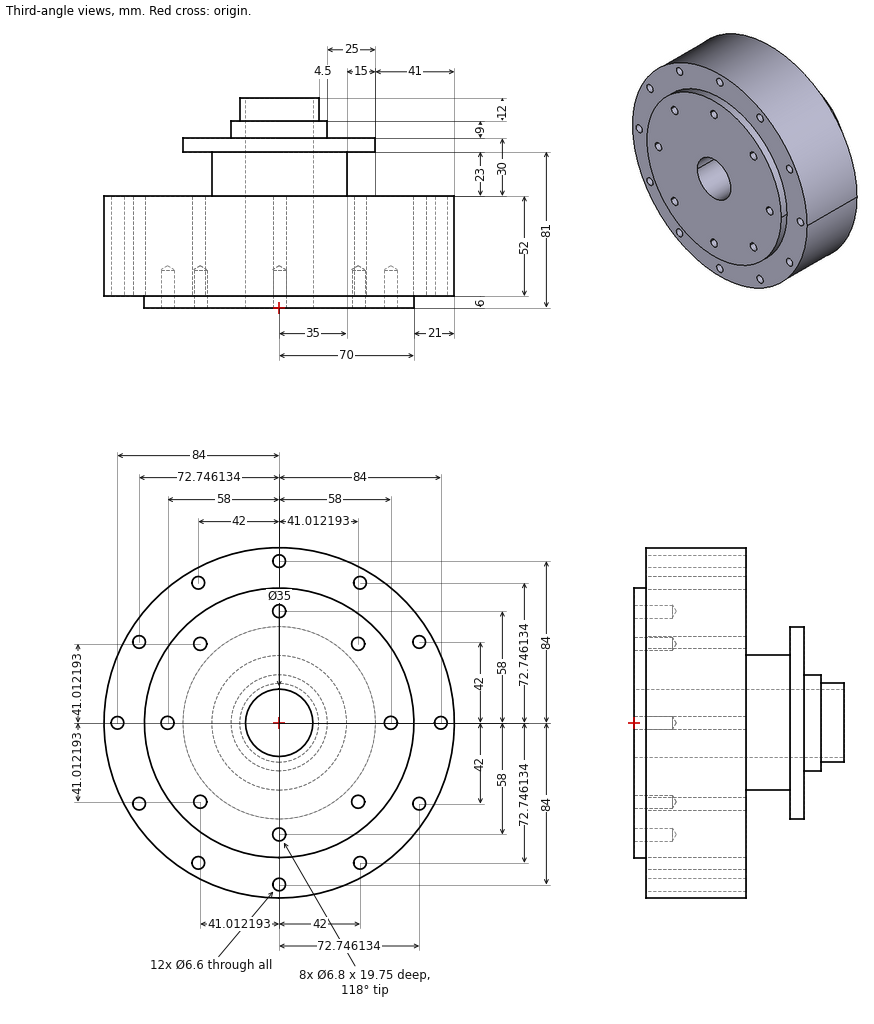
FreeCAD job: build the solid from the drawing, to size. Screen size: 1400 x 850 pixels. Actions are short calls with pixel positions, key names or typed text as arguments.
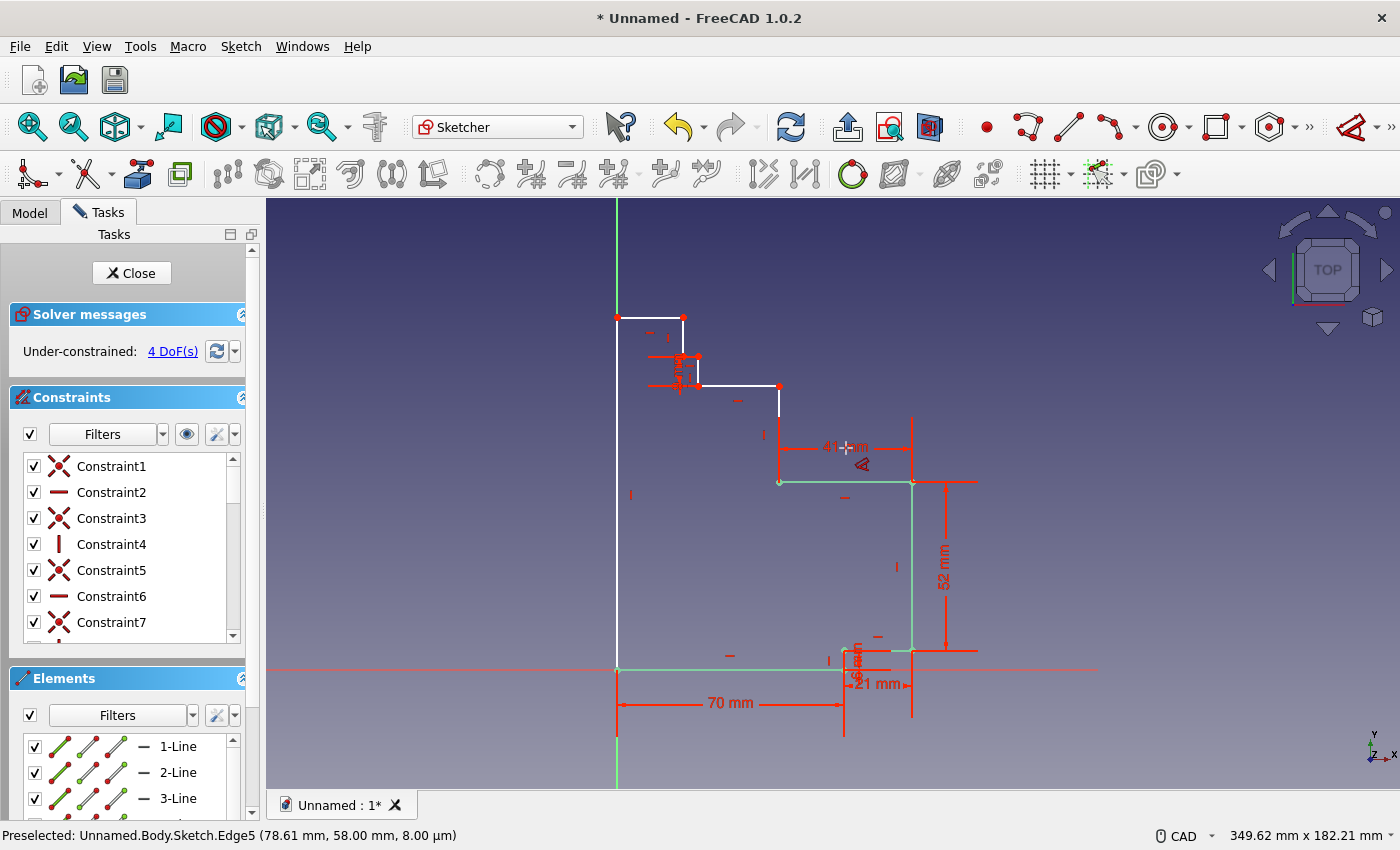
click(779, 453)
click(813, 412)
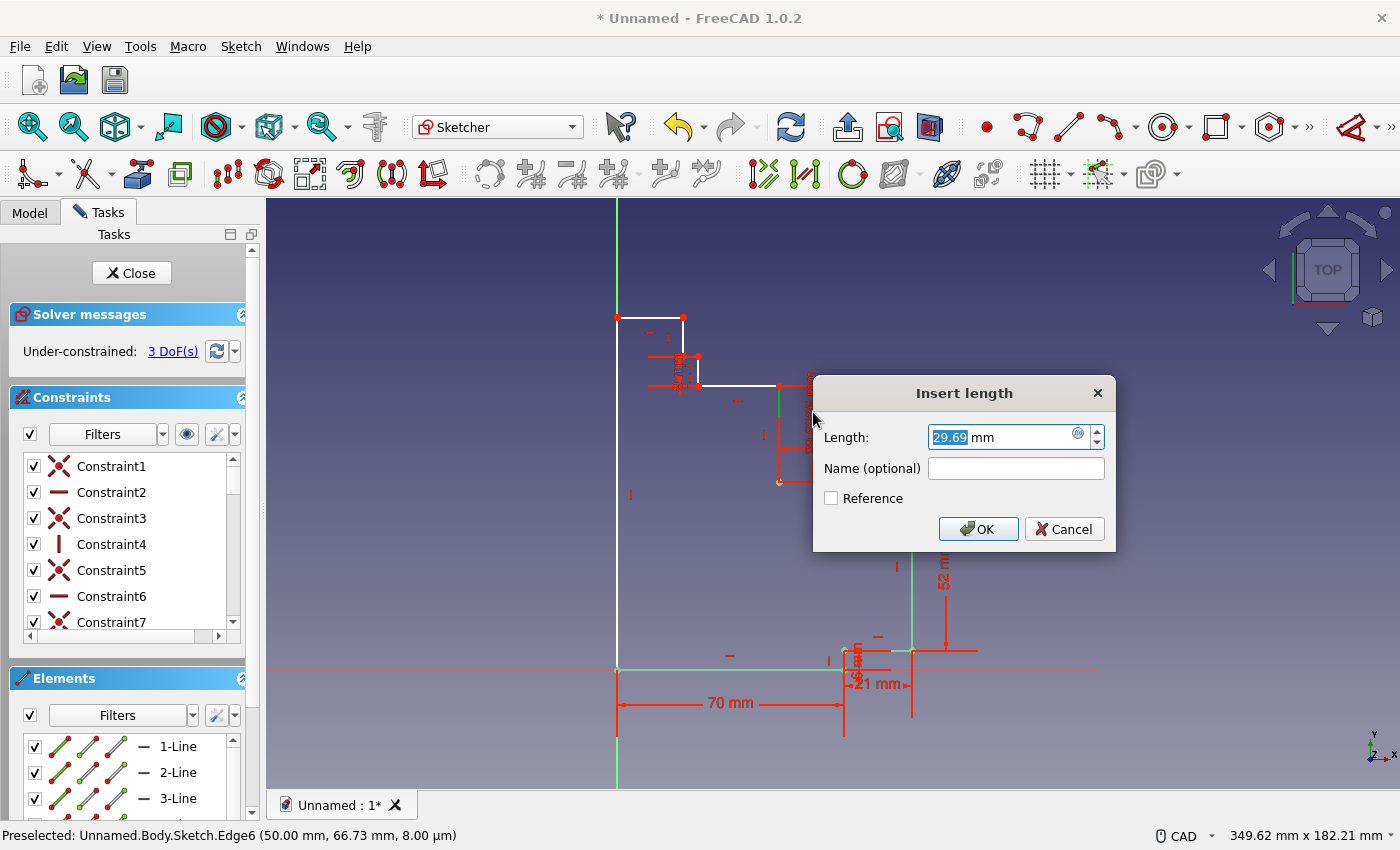
text(30)
key(Return)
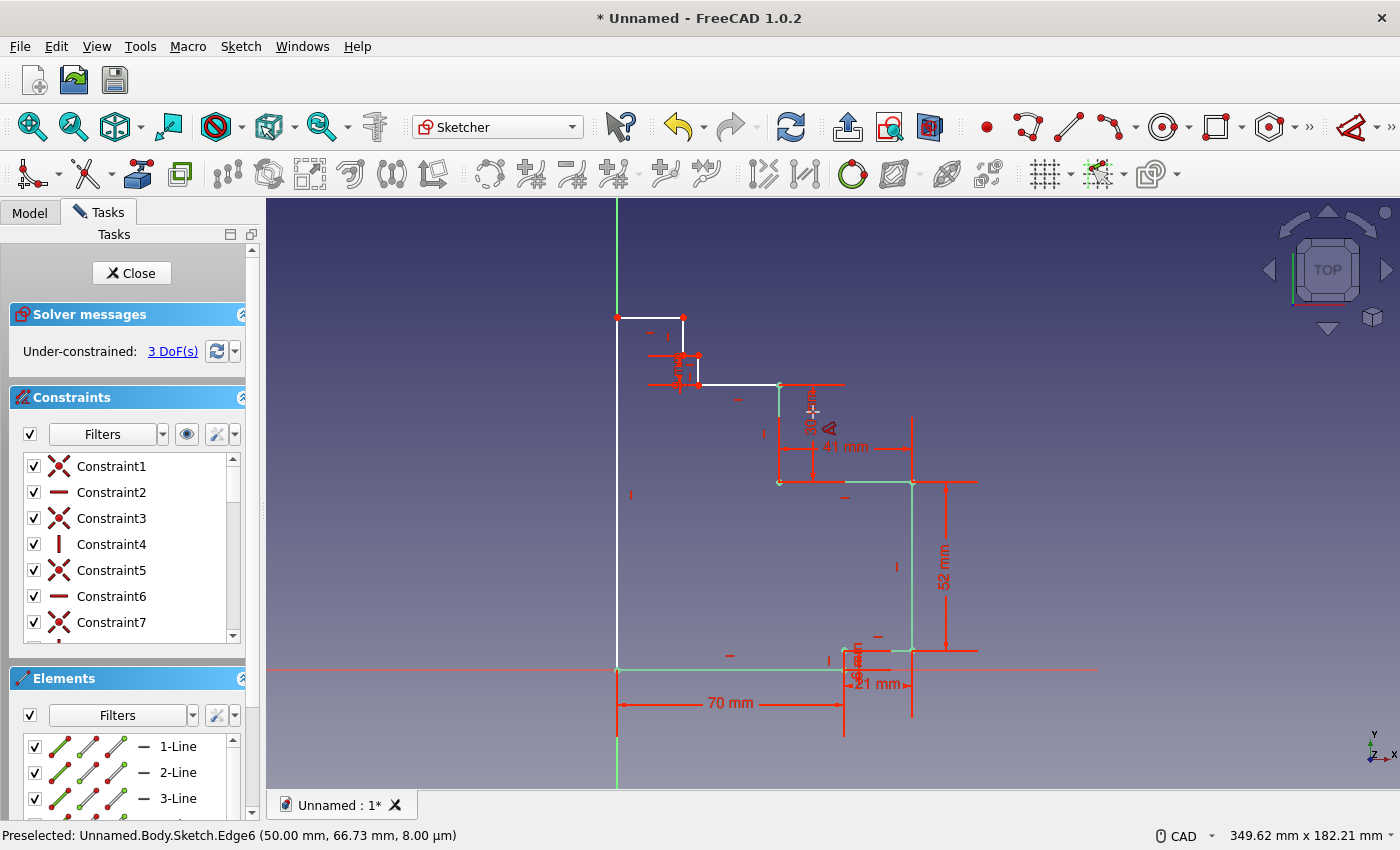
click(755, 385)
click(739, 351)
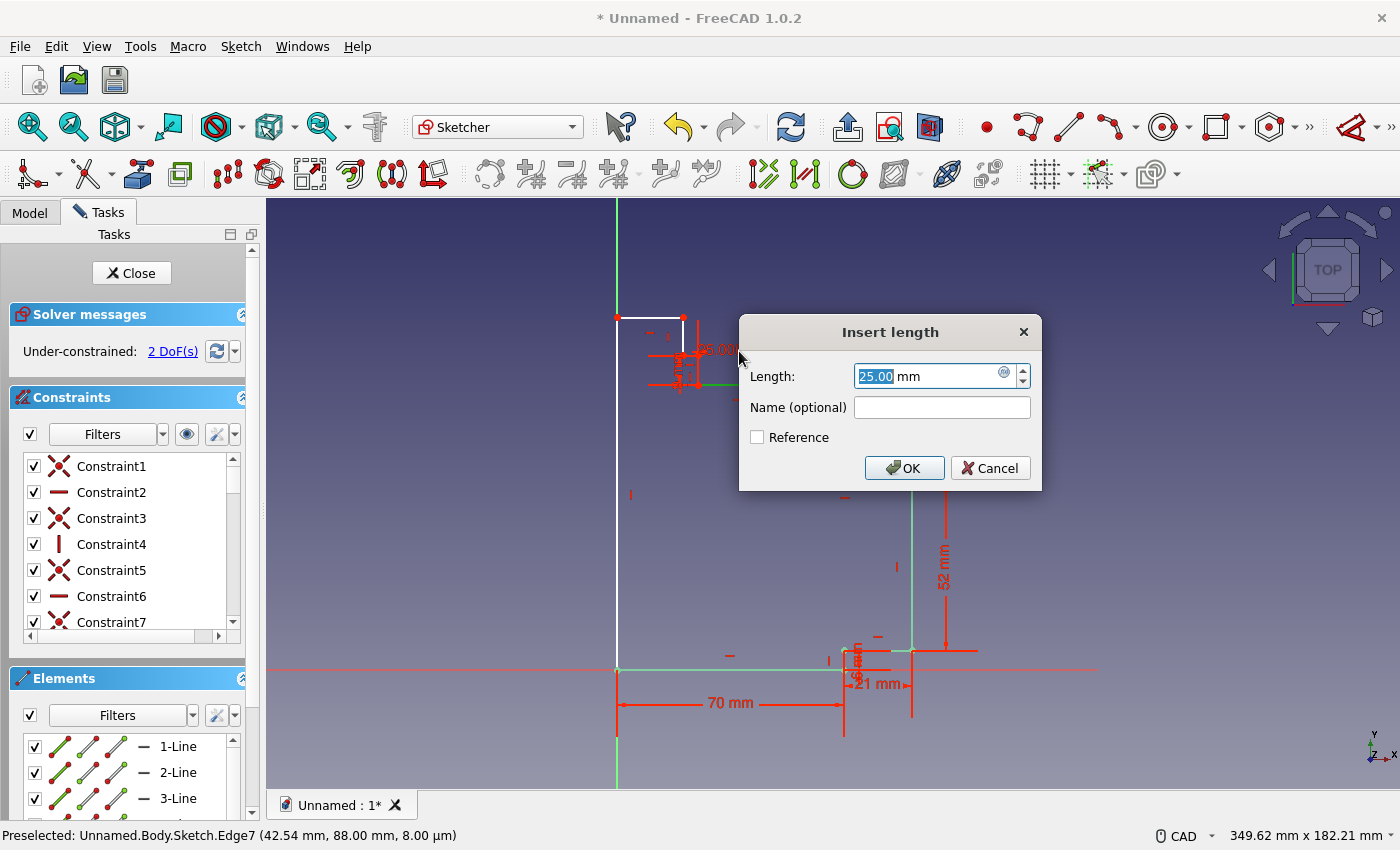
text(25)
key(Return)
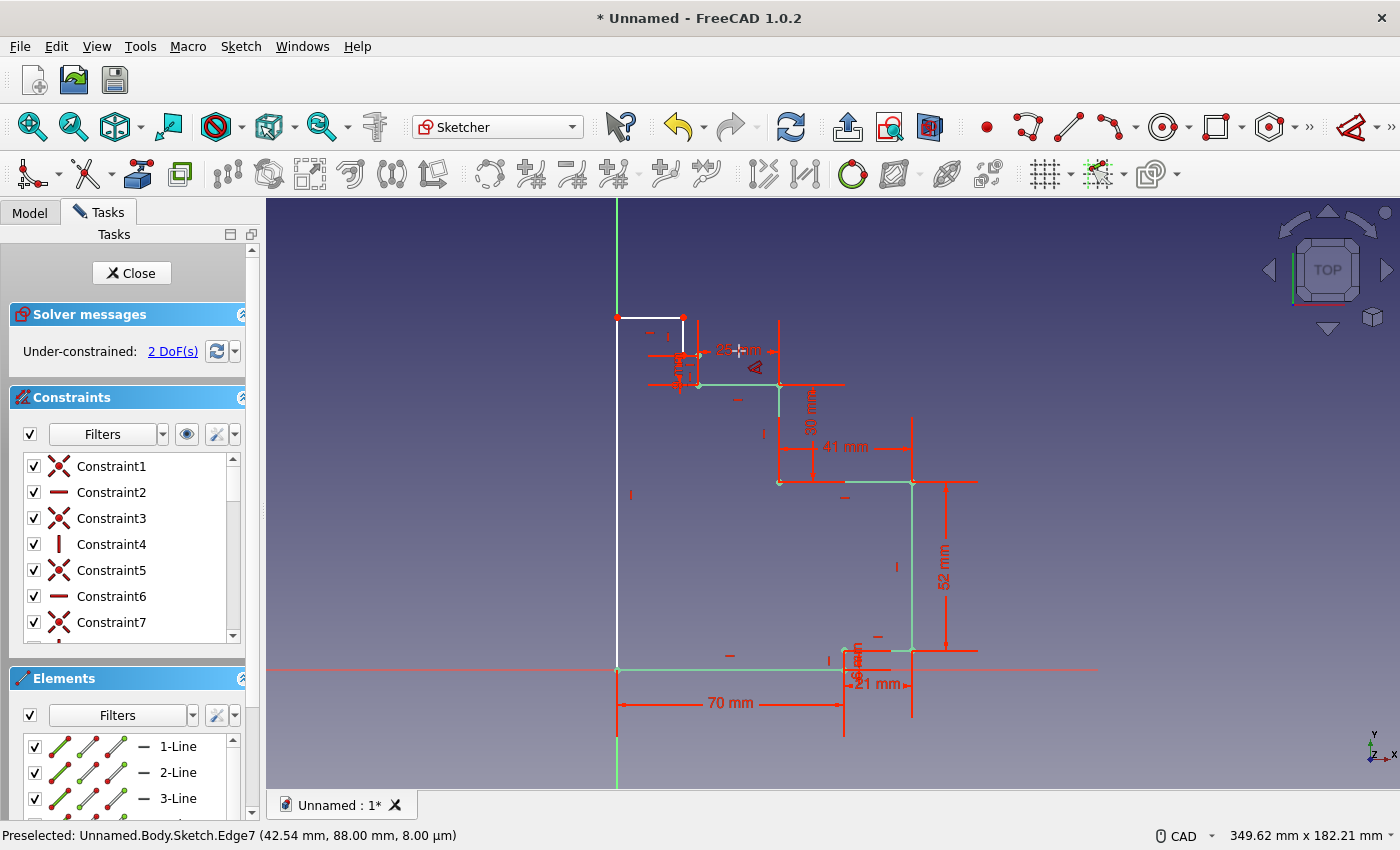
click(683, 344)
click(649, 337)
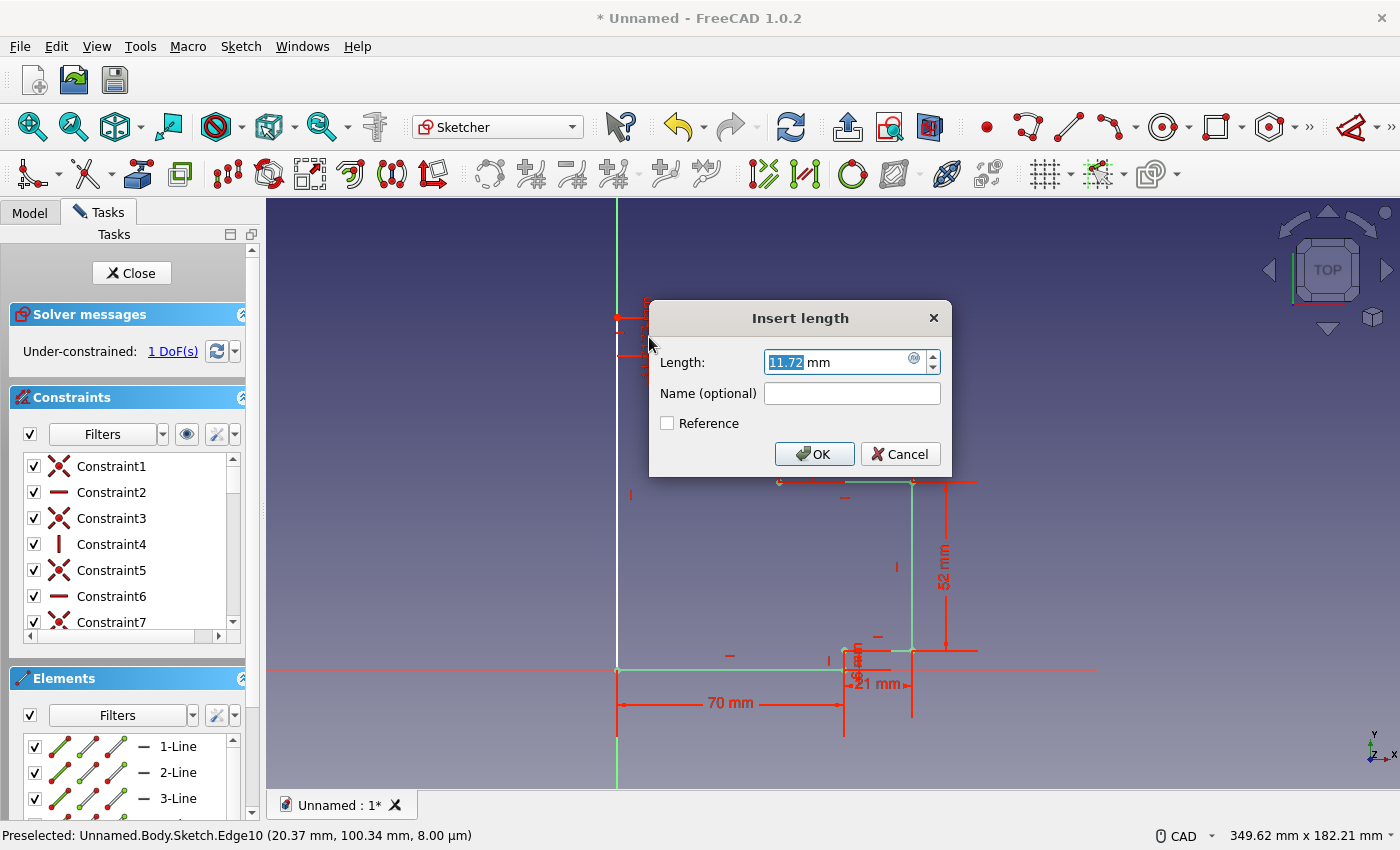
text(12)
key(Return)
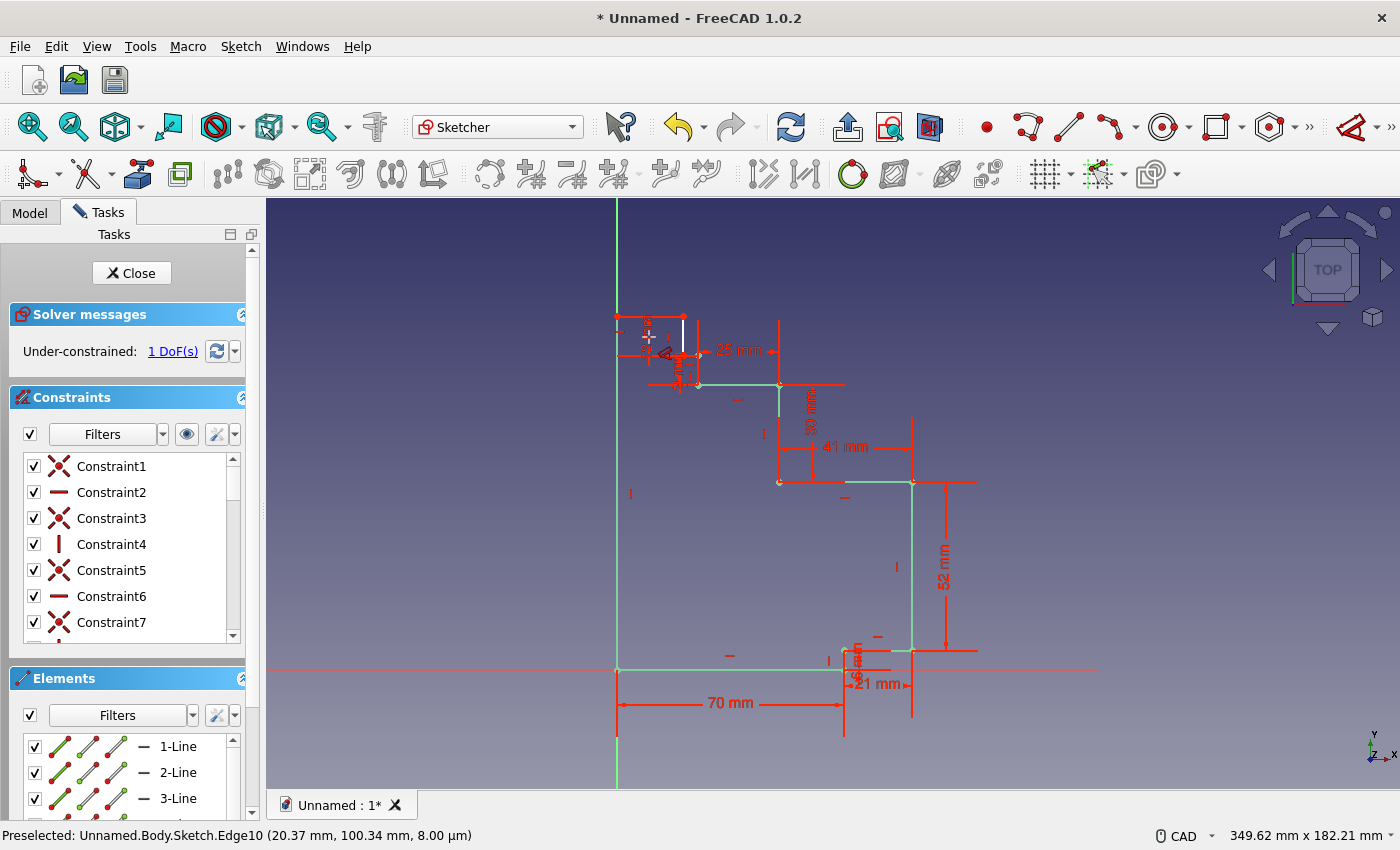
scroll(691, 356, up, 6)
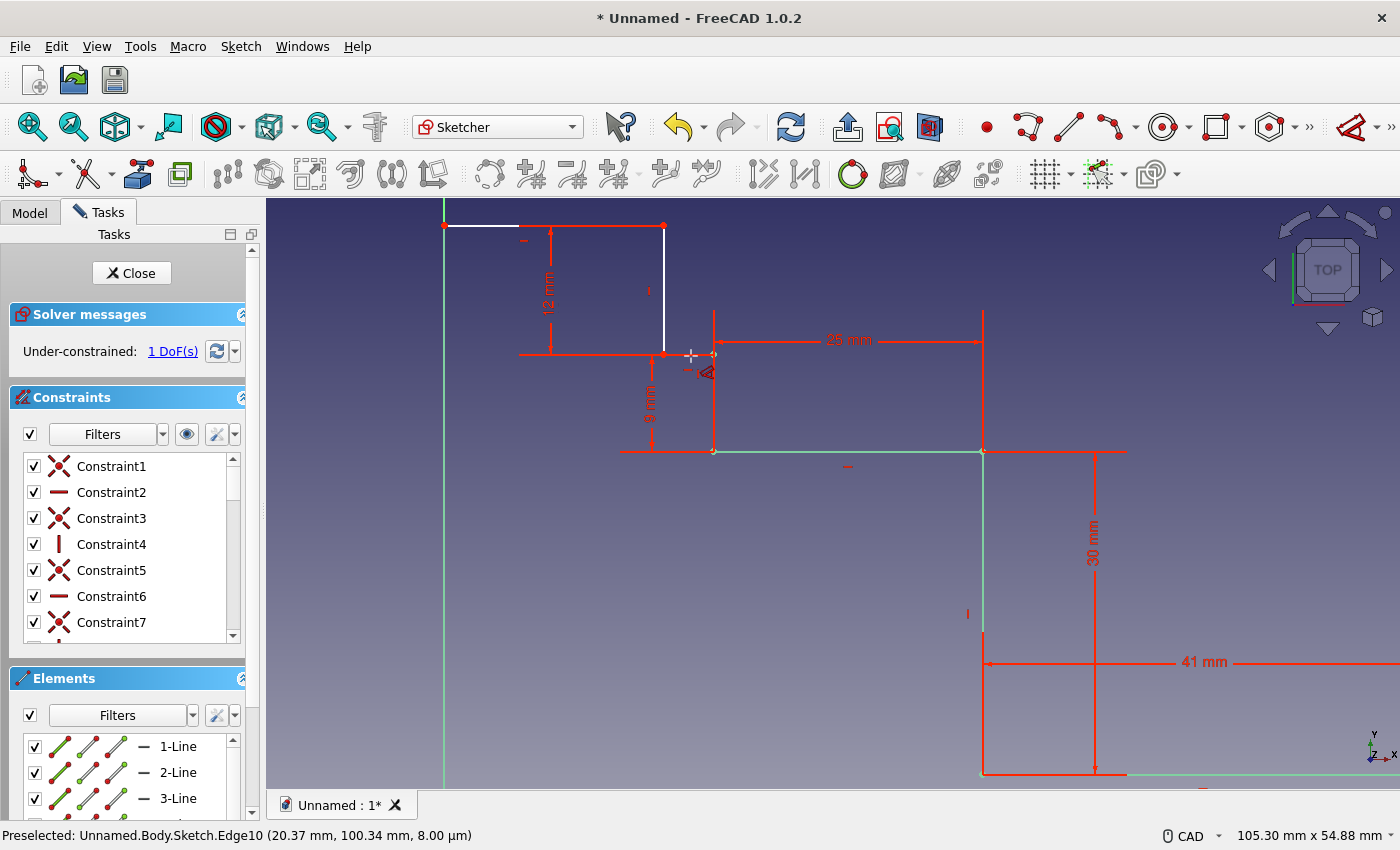
click(689, 355)
click(689, 321)